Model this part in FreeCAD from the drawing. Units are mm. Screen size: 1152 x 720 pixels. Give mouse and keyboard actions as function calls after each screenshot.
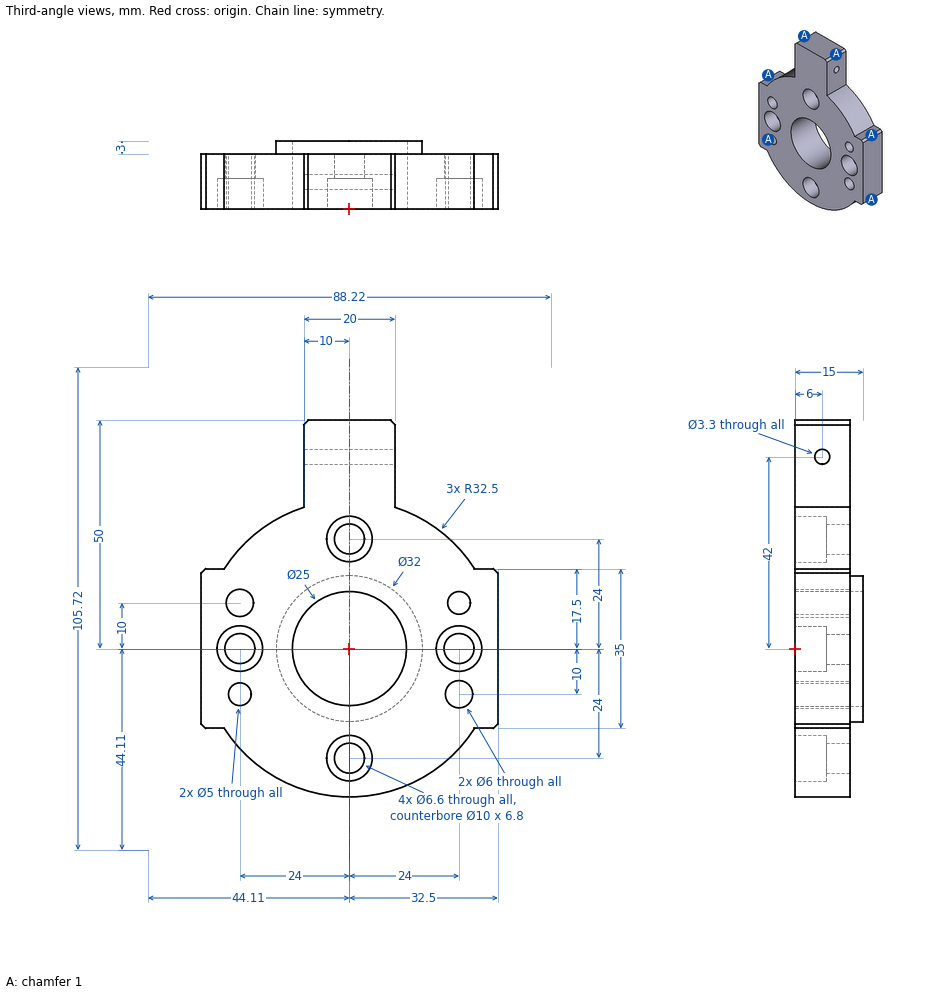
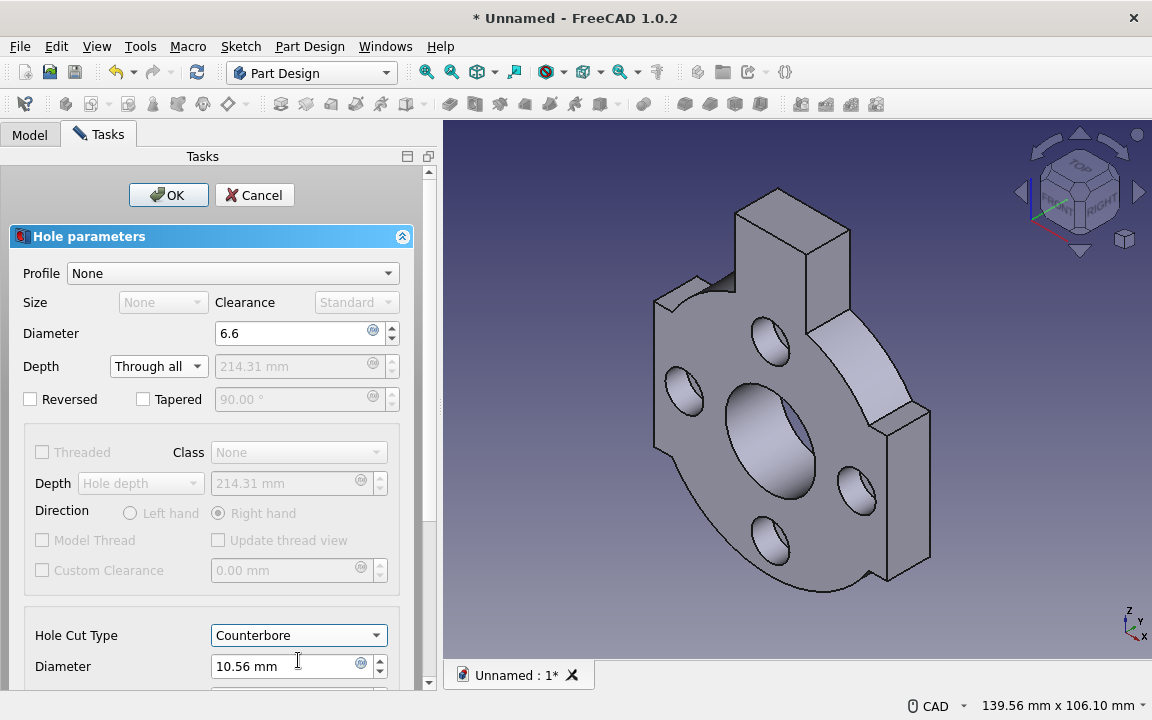
triple_click(292, 666)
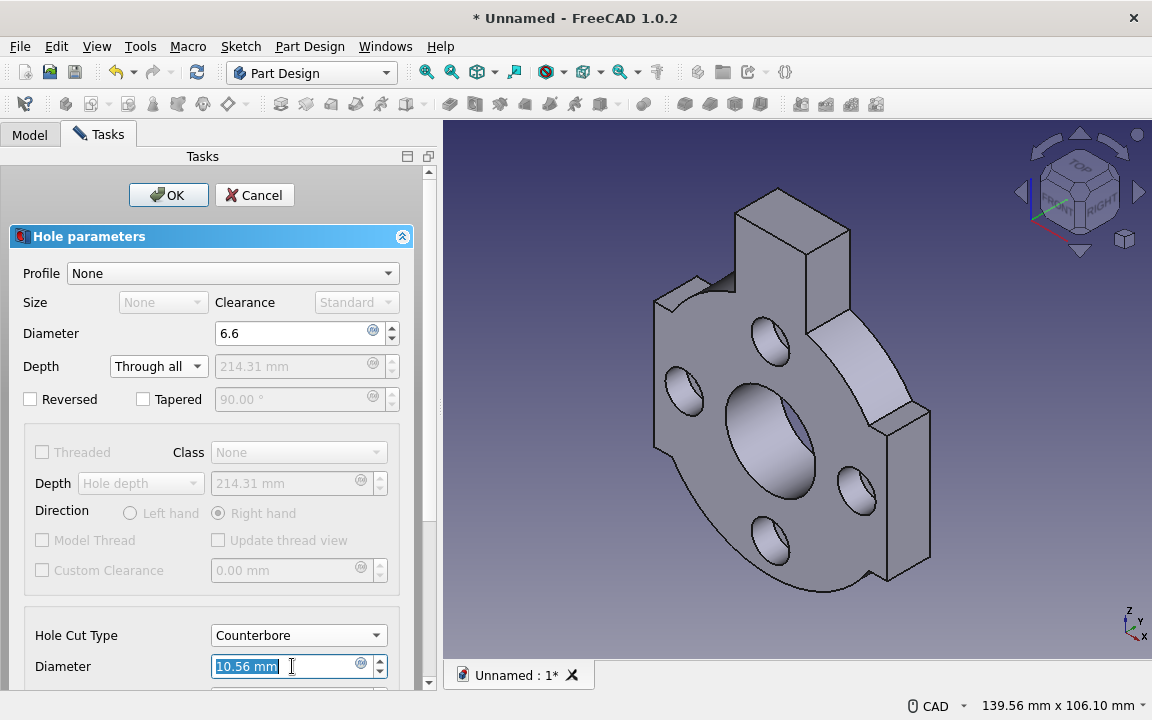
text(10)
key(Tab)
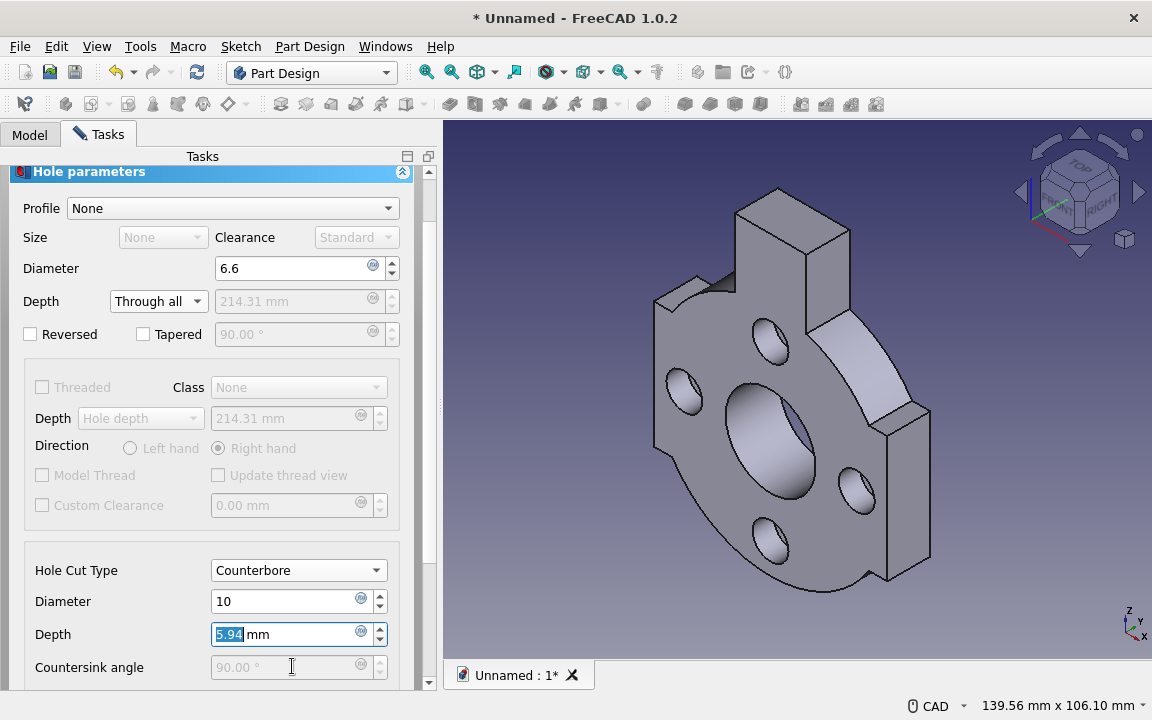
text(6.8)
key(Tab)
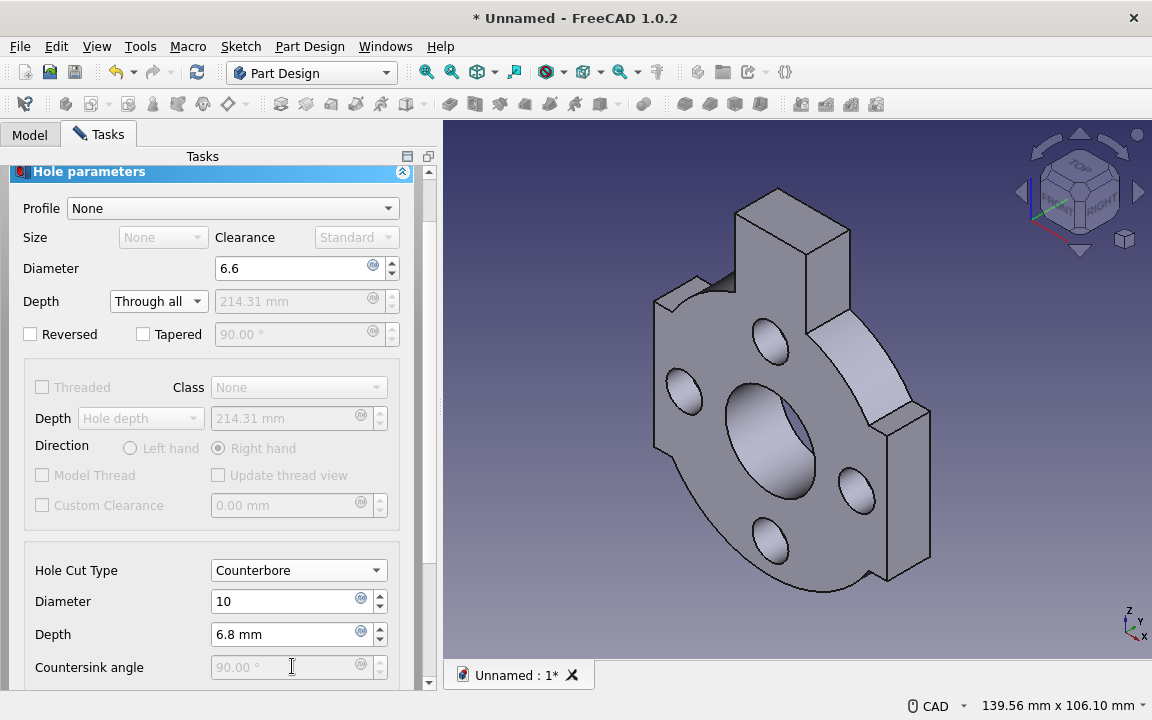
scroll(429, 428, up, 2)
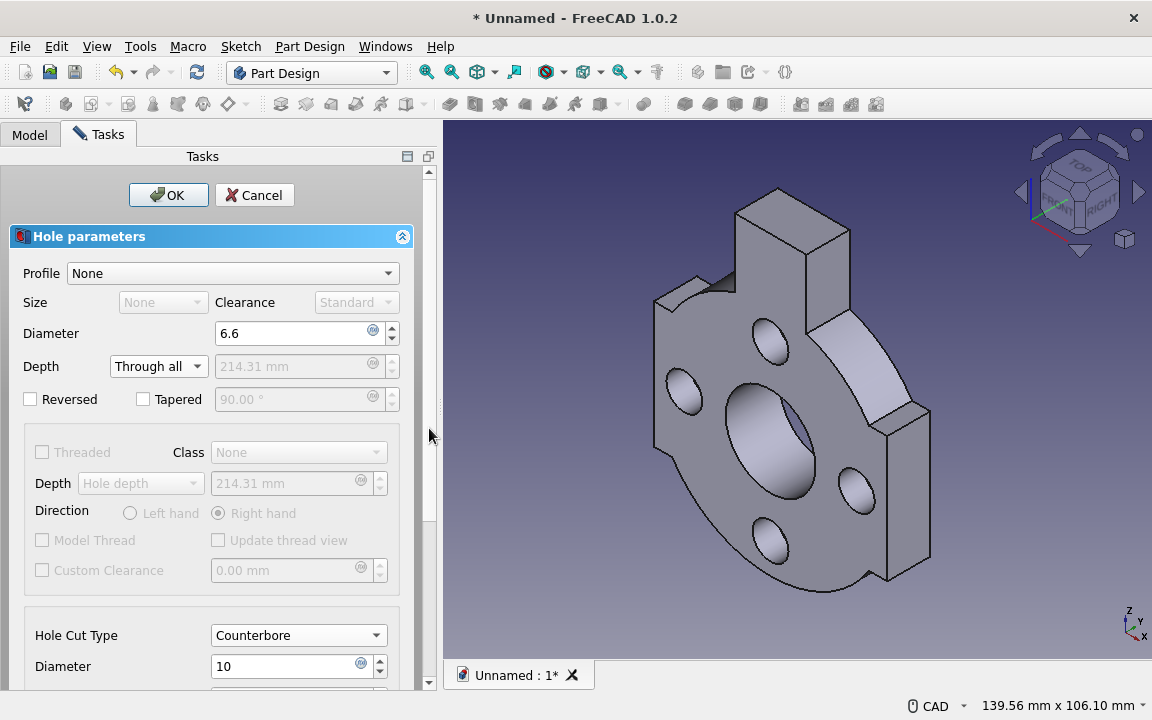
click(169, 195)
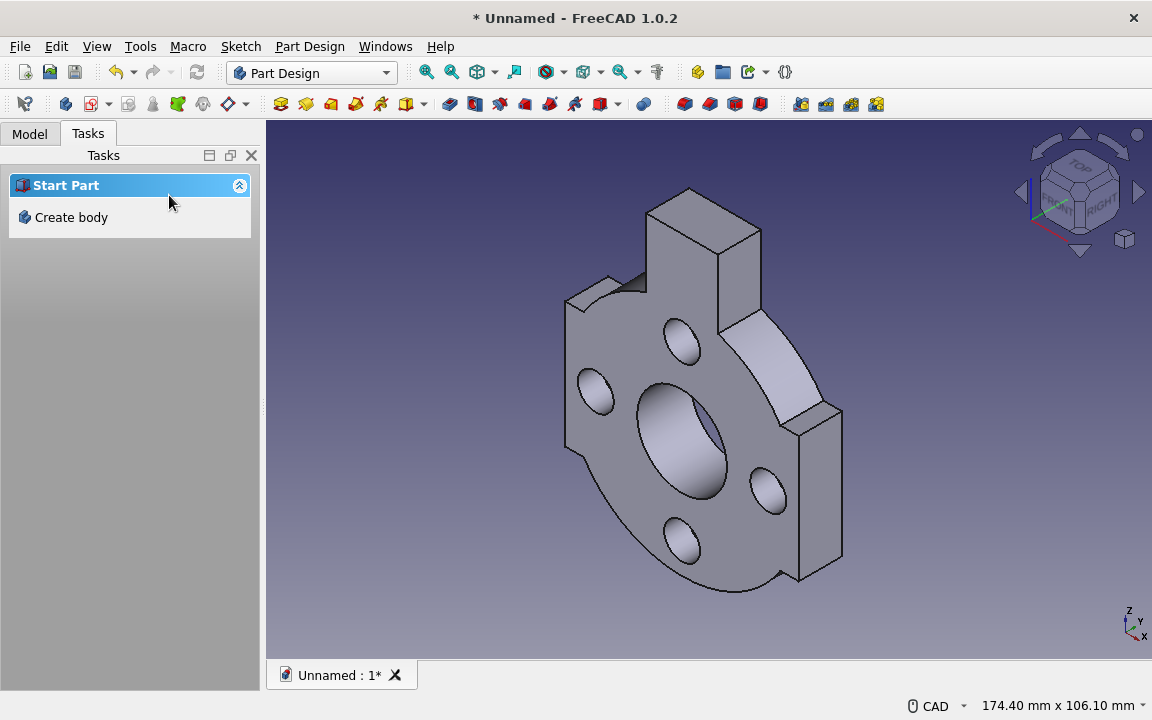
click(90, 104)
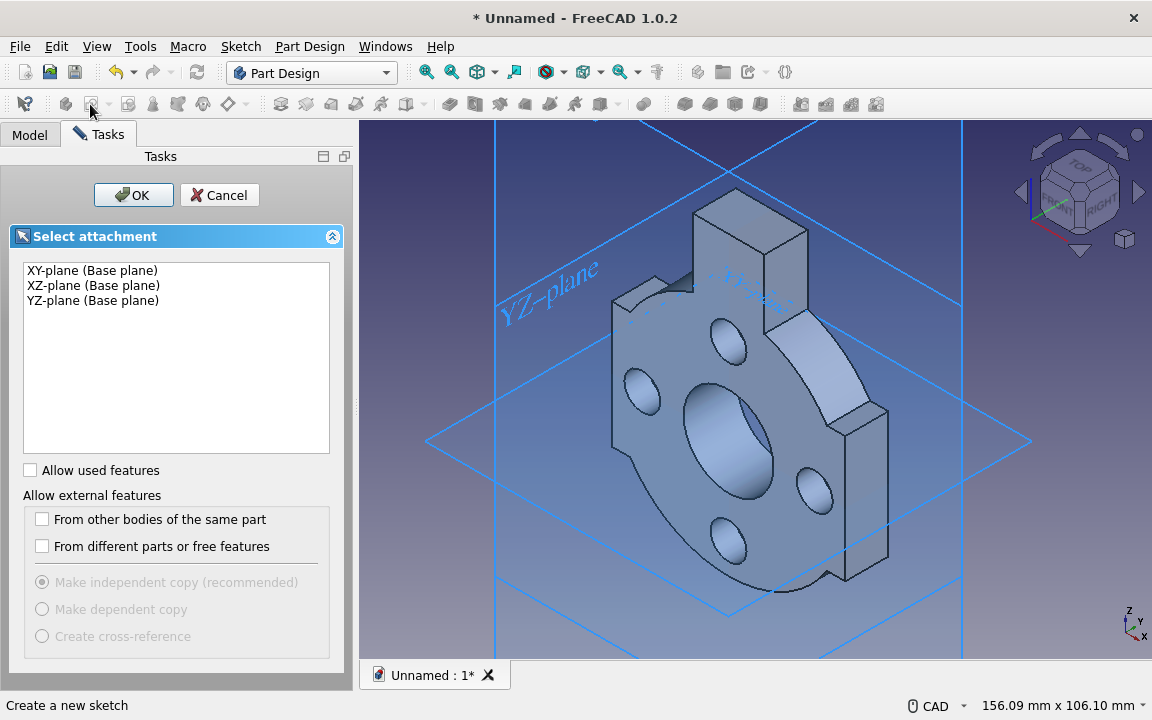
click(84, 286)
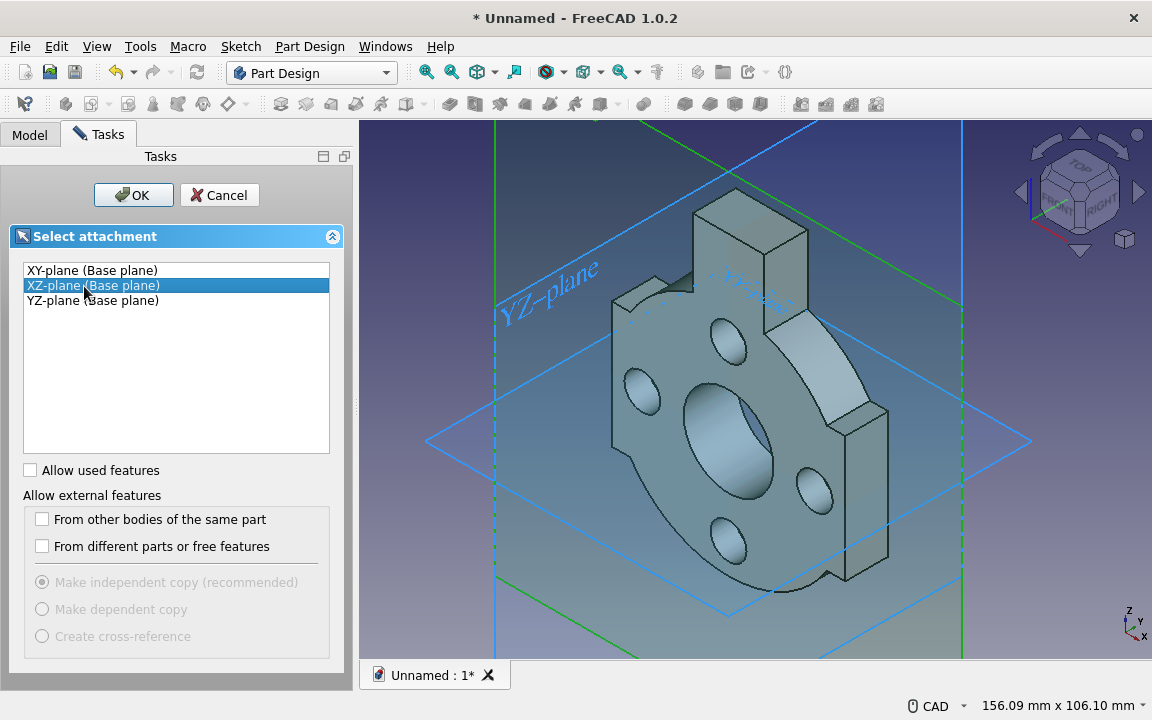
click(134, 195)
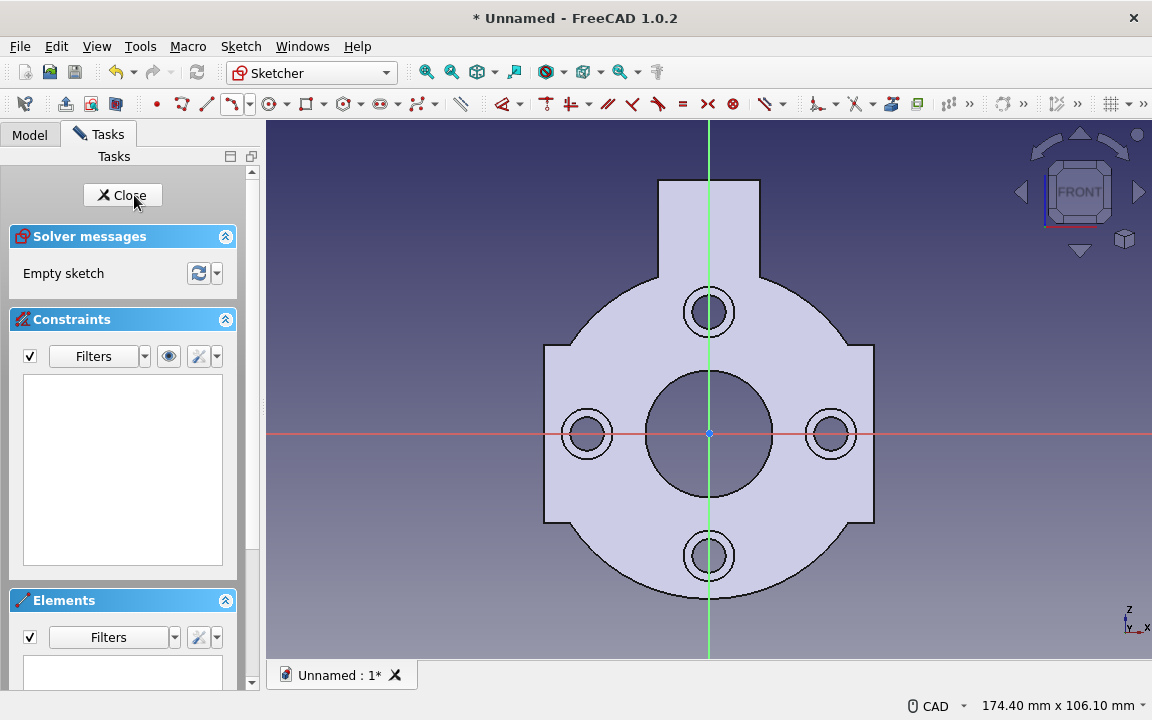
scroll(792, 488, up, 3)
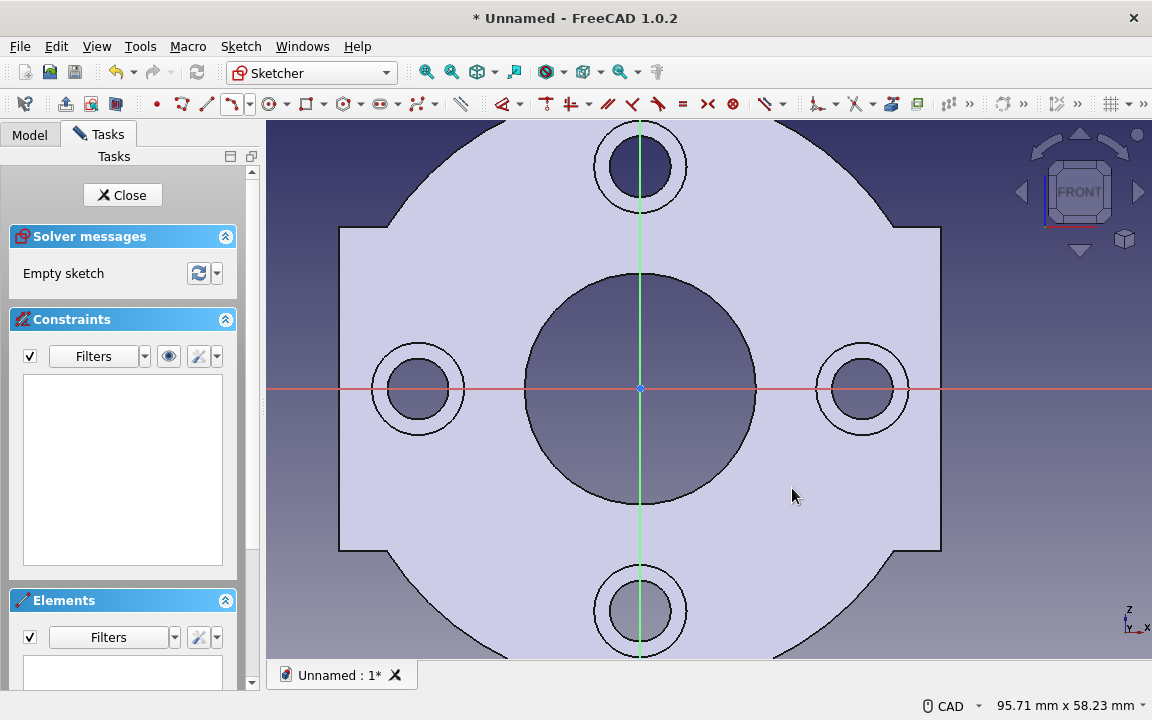
click(268, 104)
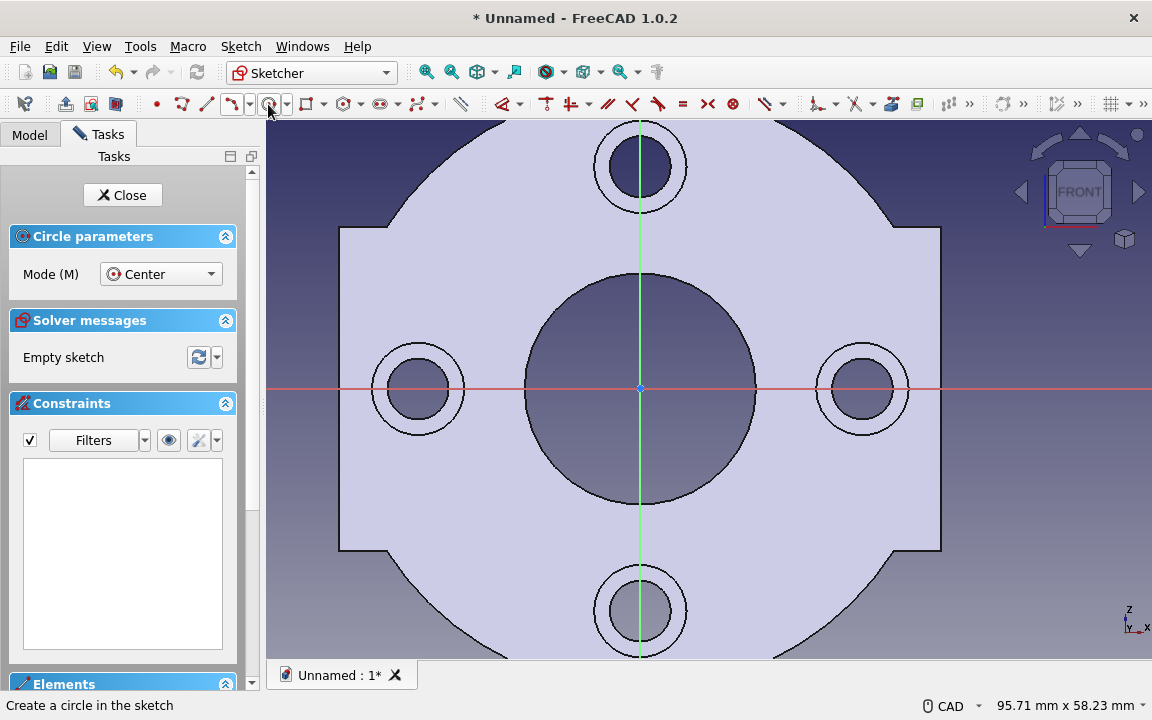
click(862, 482)
click(882, 462)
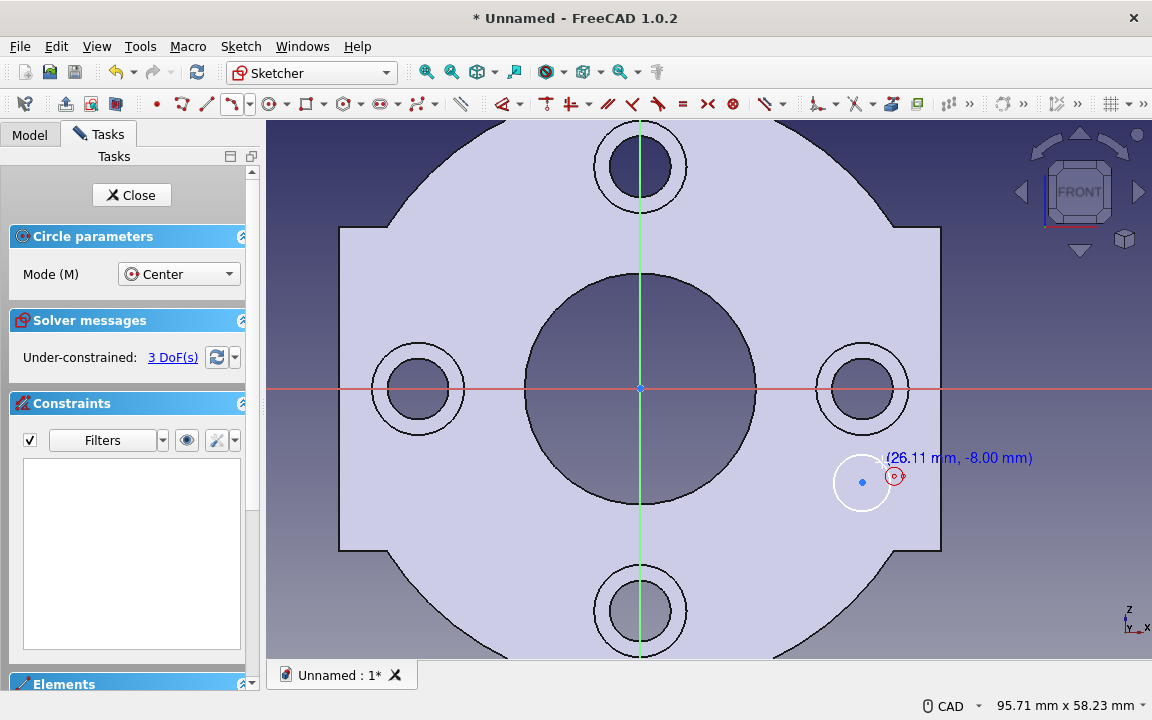
click(418, 296)
click(438, 277)
key(Escape)